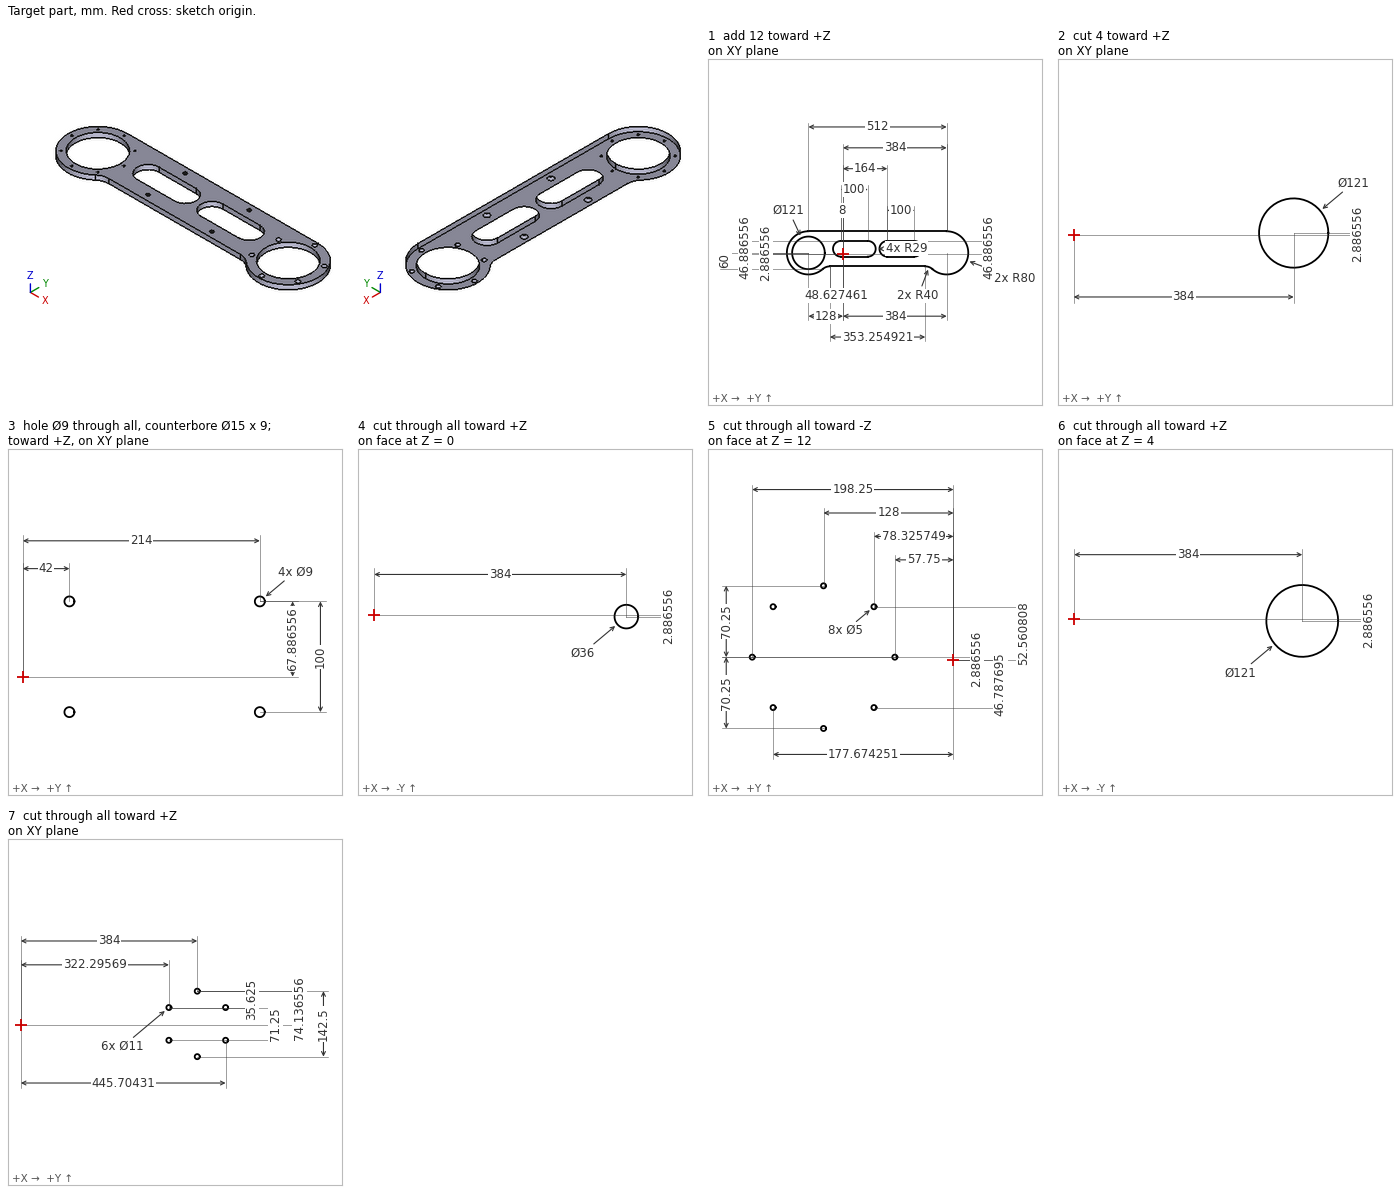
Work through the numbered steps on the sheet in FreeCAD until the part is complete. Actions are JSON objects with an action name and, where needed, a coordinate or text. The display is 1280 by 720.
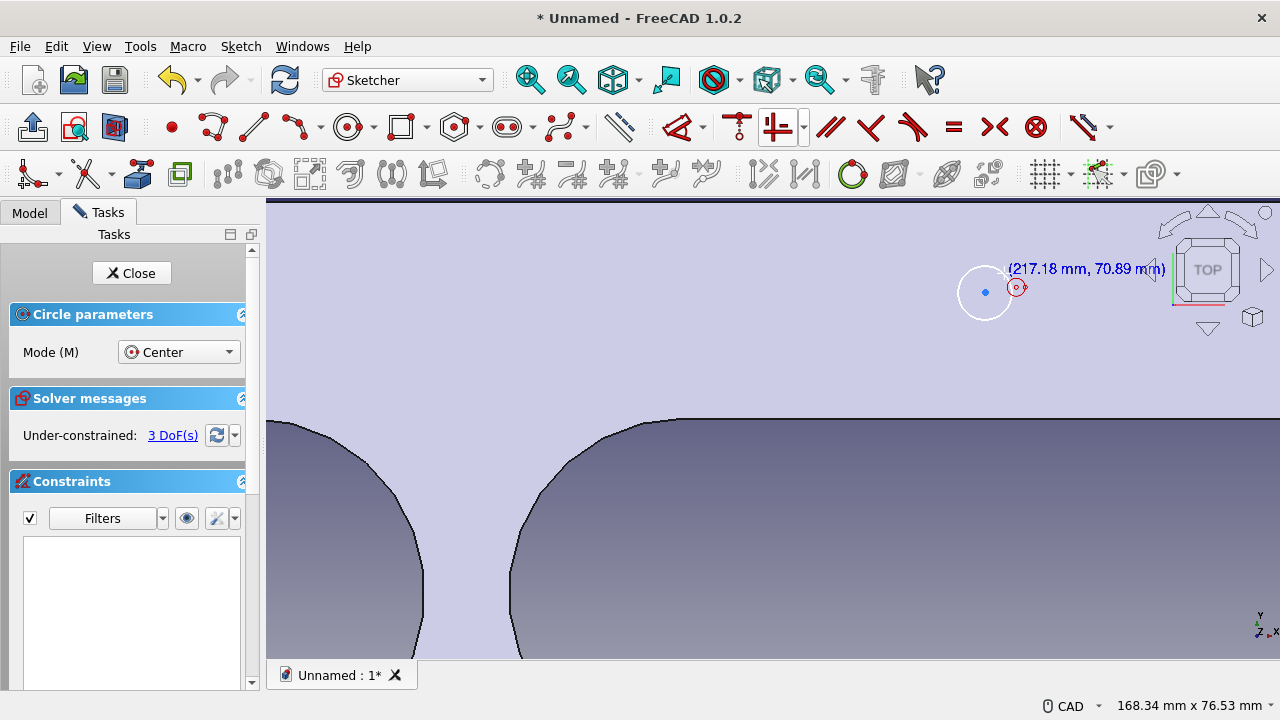
{"action": "scroll", "coordinate": [991, 294], "scroll_direction": "down", "scroll_amount": 4}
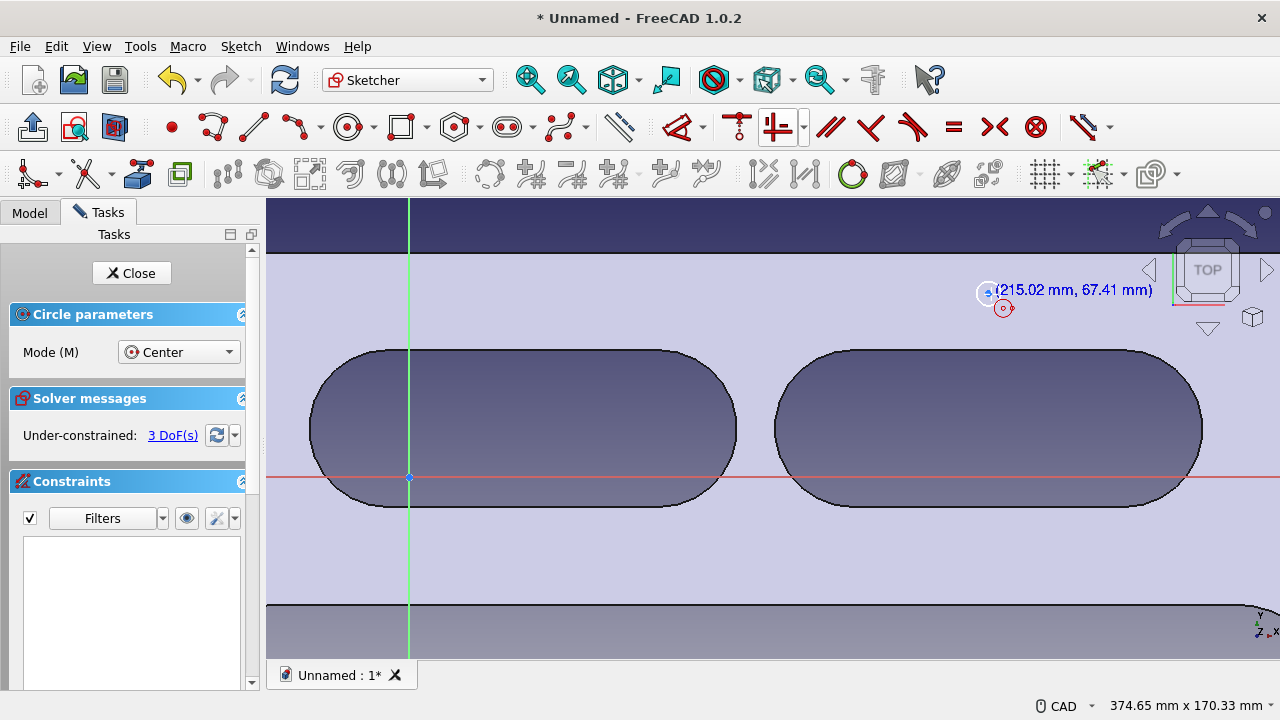
{"action": "scroll", "coordinate": [989, 564], "scroll_direction": "up", "scroll_amount": 4}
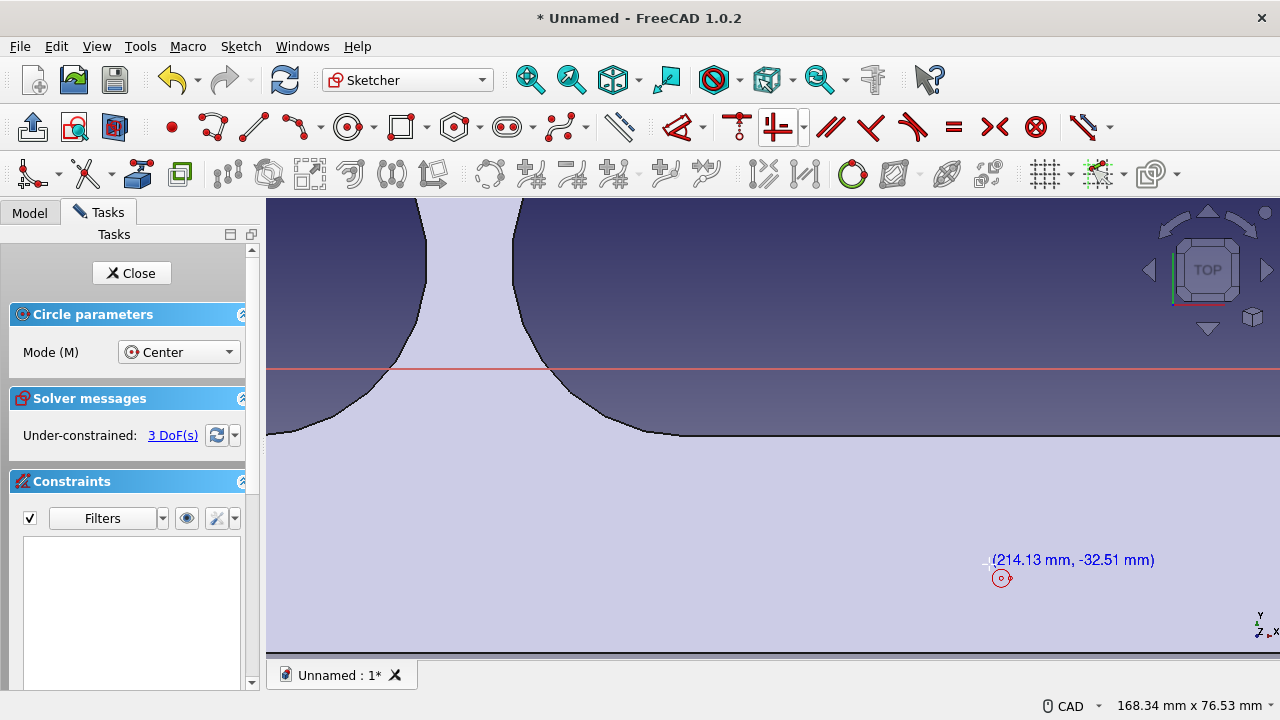
{"action": "left_click", "coordinate": [987, 563]}
{"action": "left_click", "coordinate": [1006, 544]}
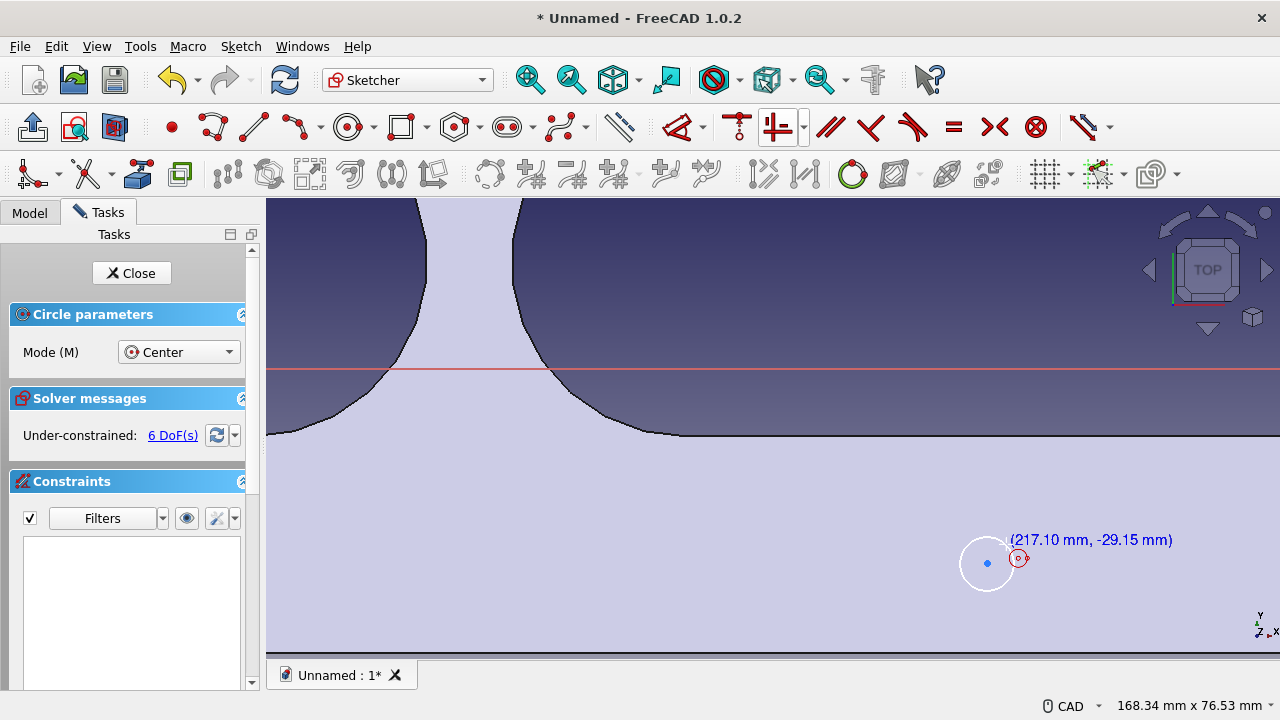
{"action": "scroll", "coordinate": [989, 565], "scroll_direction": "down", "scroll_amount": 4}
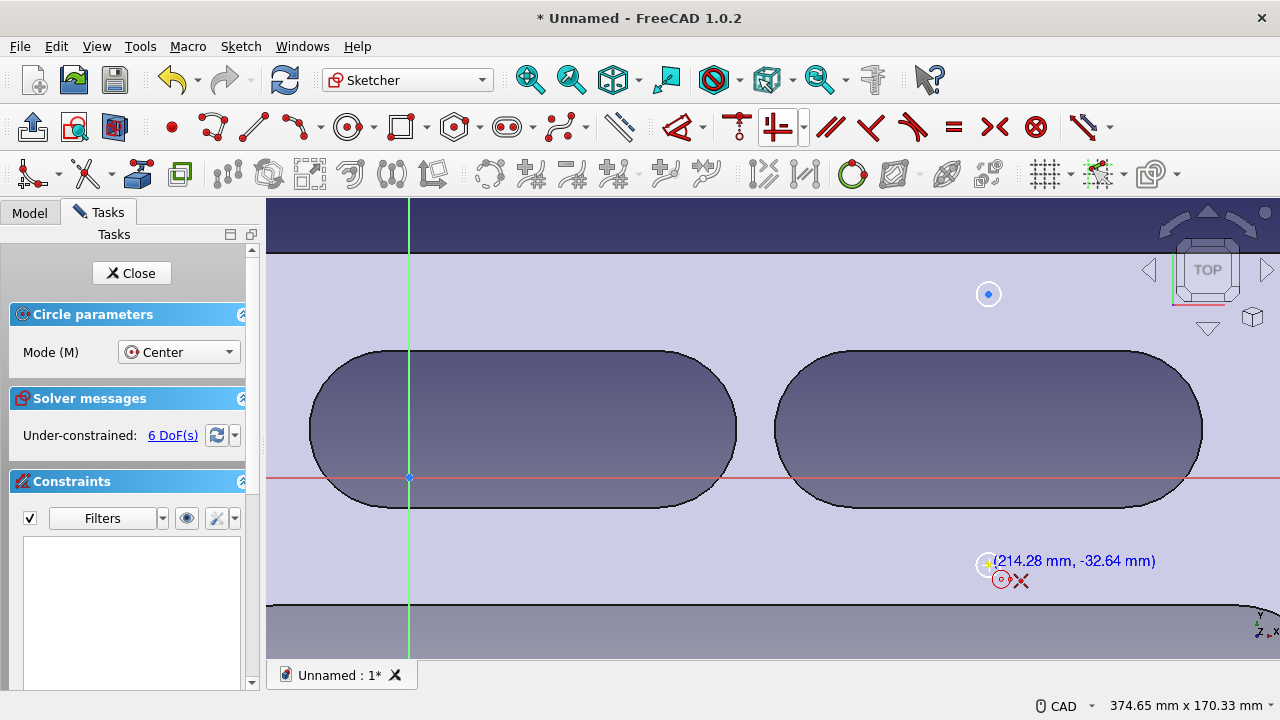
{"action": "scroll", "coordinate": [523, 294], "scroll_direction": "up", "scroll_amount": 4}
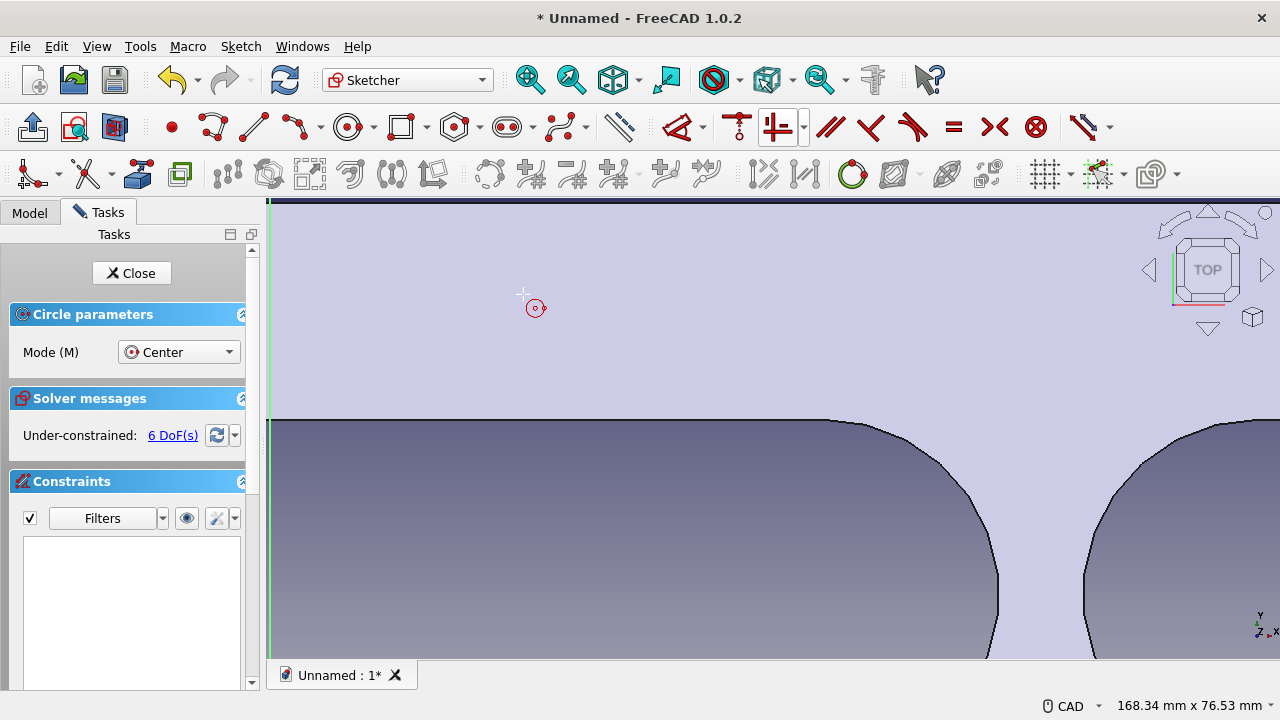
{"action": "left_click", "coordinate": [523, 293]}
{"action": "left_click", "coordinate": [542, 274]}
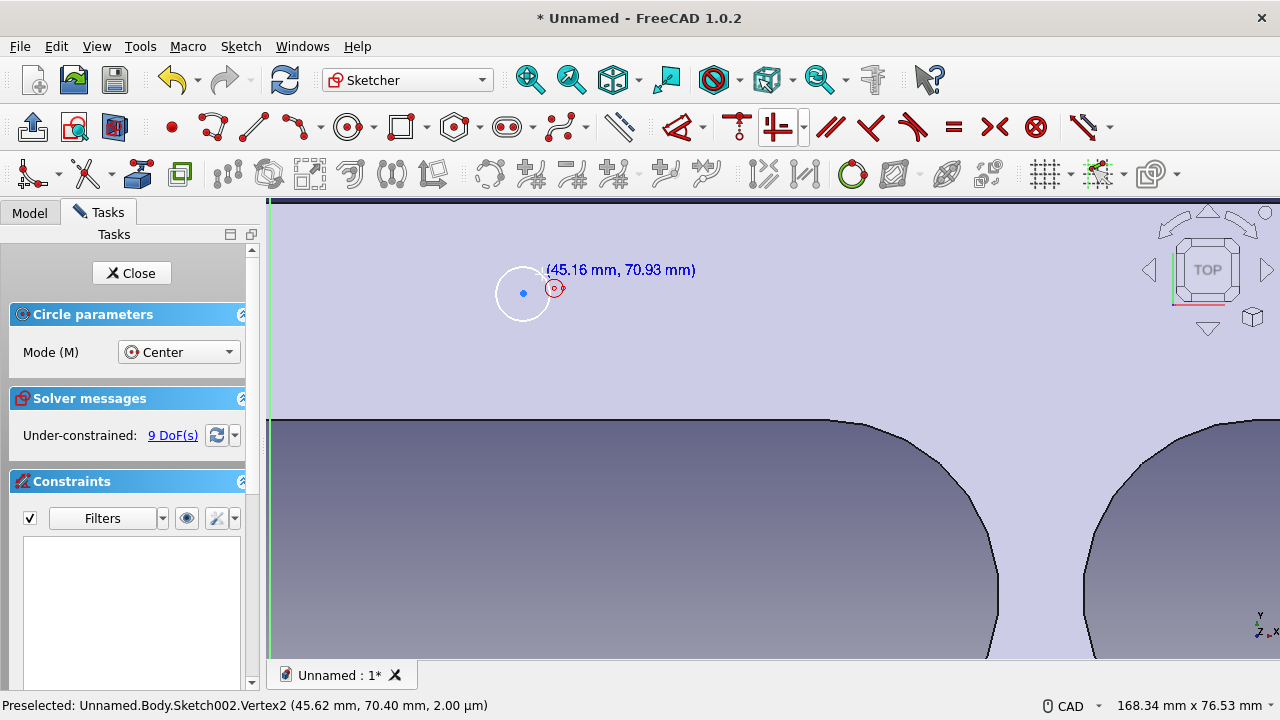
{"action": "scroll", "coordinate": [522, 293], "scroll_direction": "down", "scroll_amount": 4}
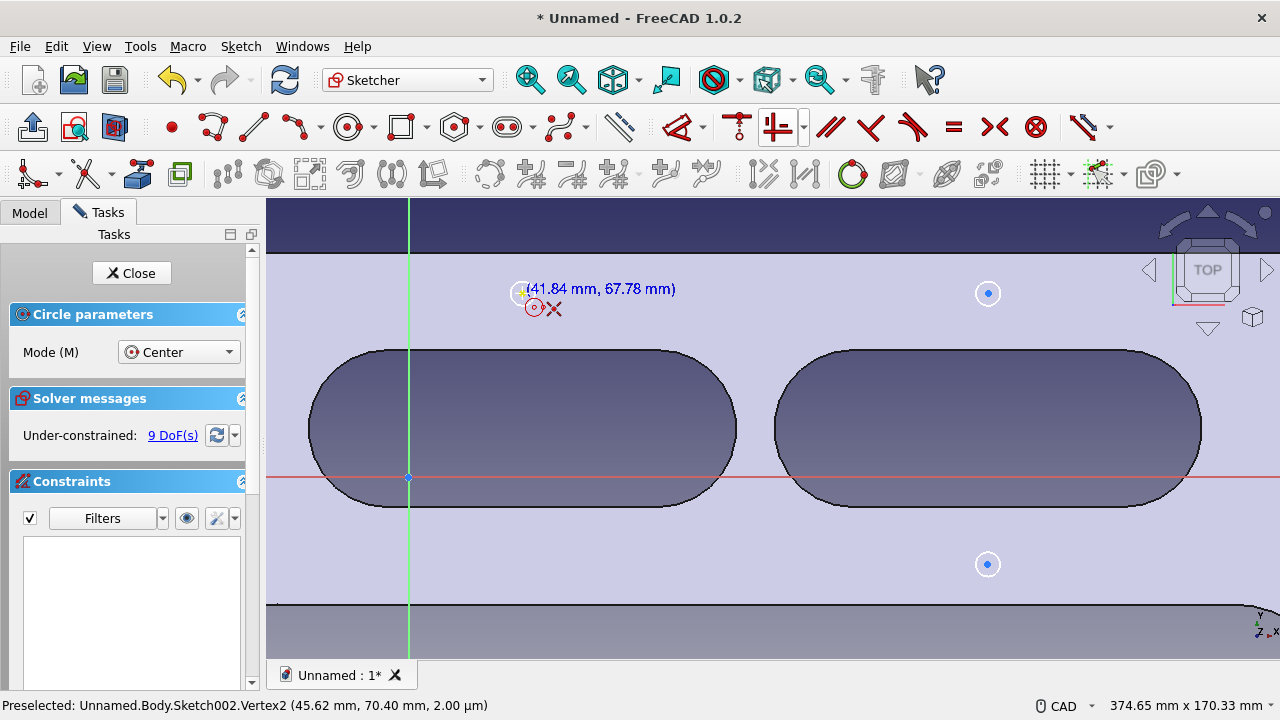
{"action": "scroll", "coordinate": [523, 564], "scroll_direction": "up", "scroll_amount": 4}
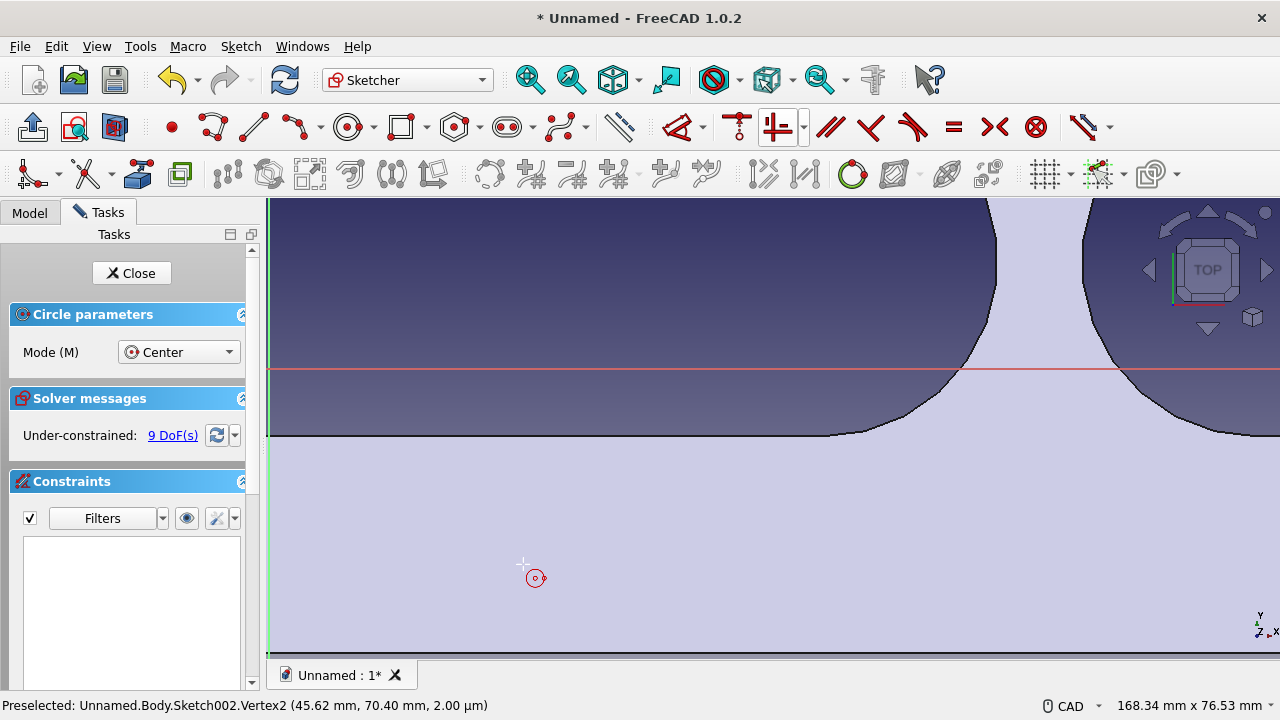
{"action": "left_click", "coordinate": [522, 563]}
{"action": "left_click", "coordinate": [541, 544]}
{"action": "key", "text": "Escape"}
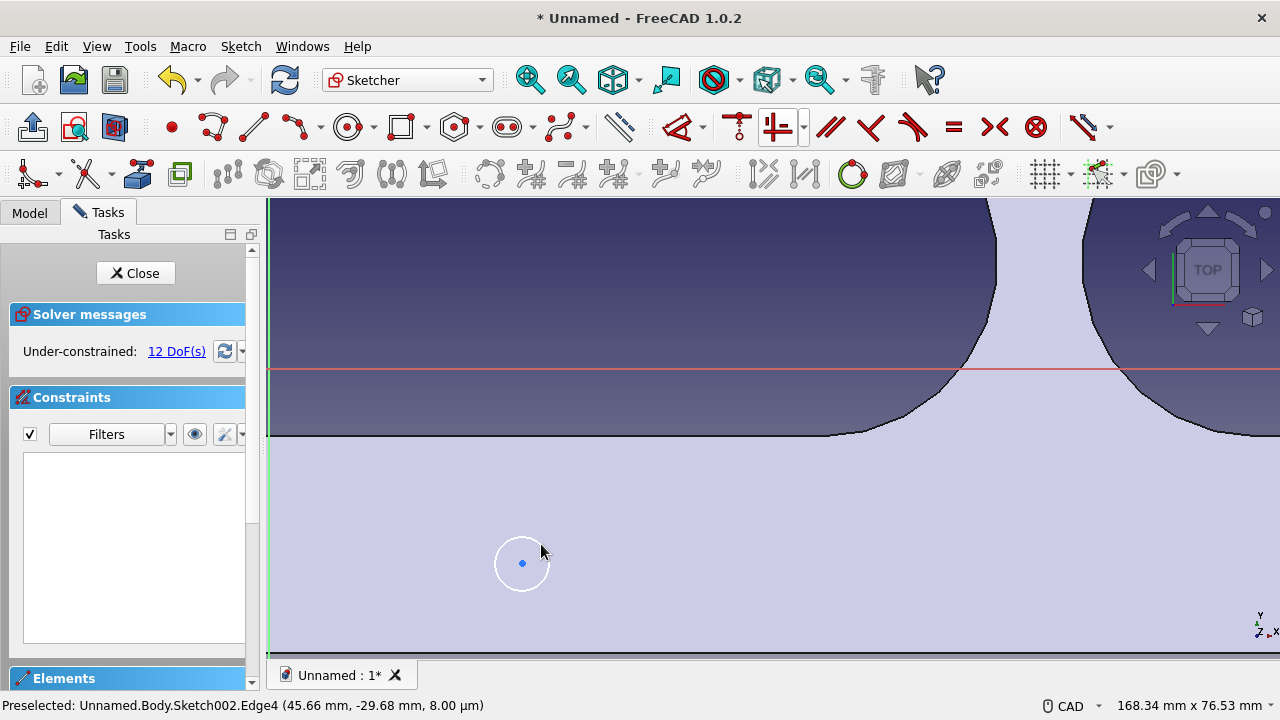
{"action": "scroll", "coordinate": [523, 565], "scroll_direction": "down", "scroll_amount": 4}